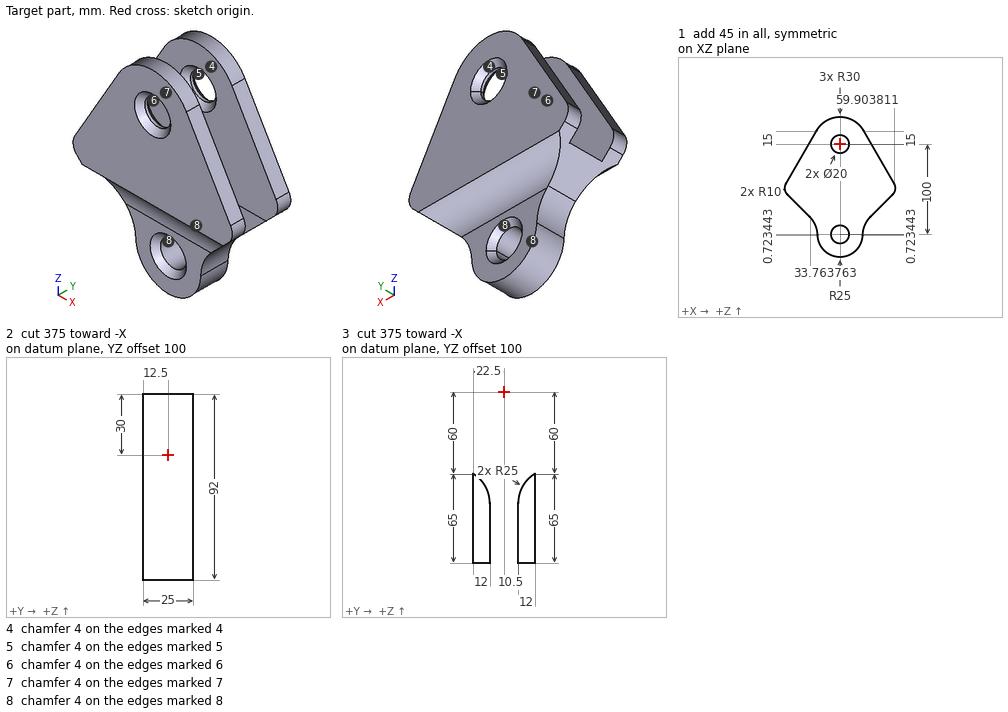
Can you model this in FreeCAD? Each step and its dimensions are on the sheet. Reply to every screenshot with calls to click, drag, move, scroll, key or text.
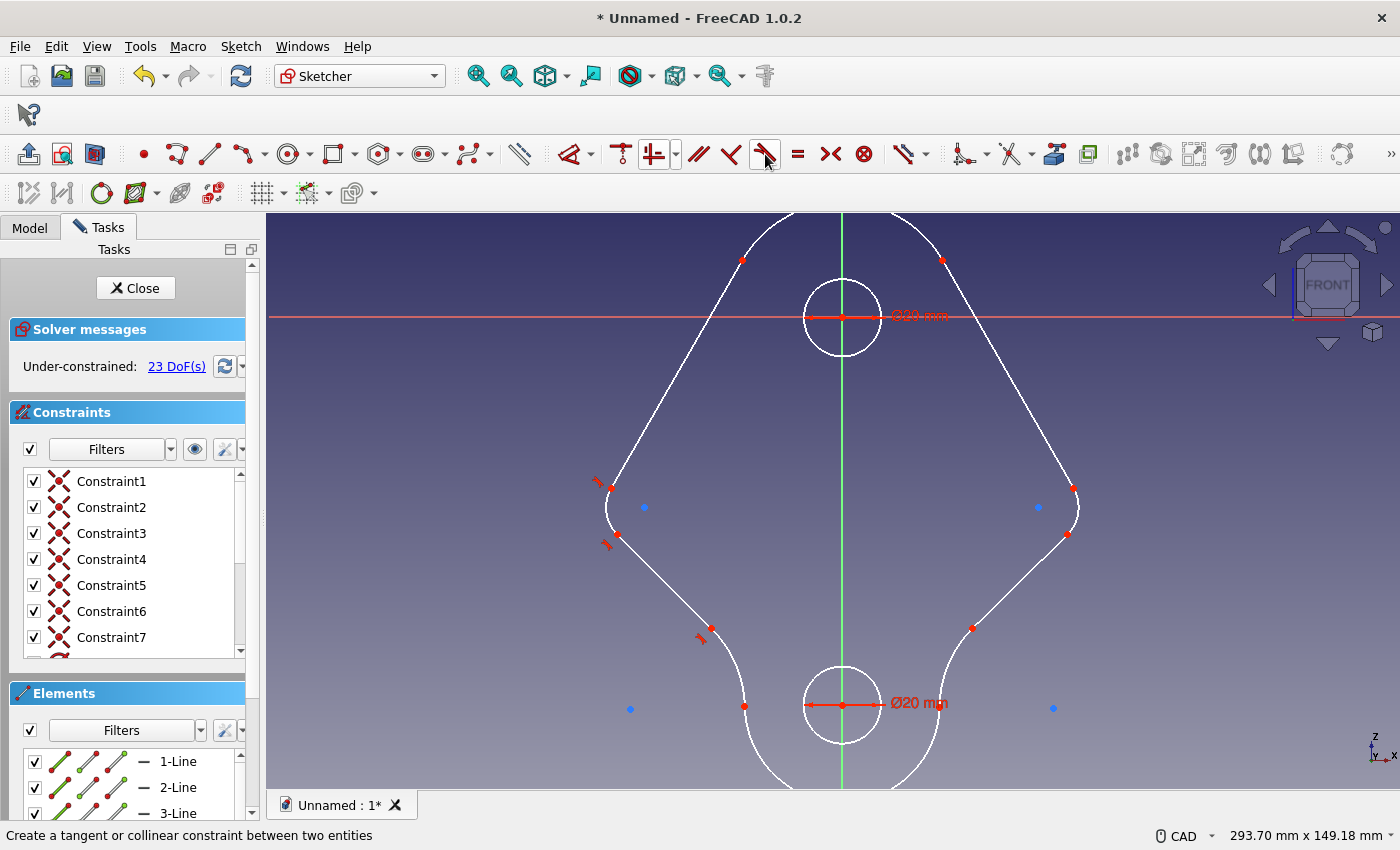
click(651, 420)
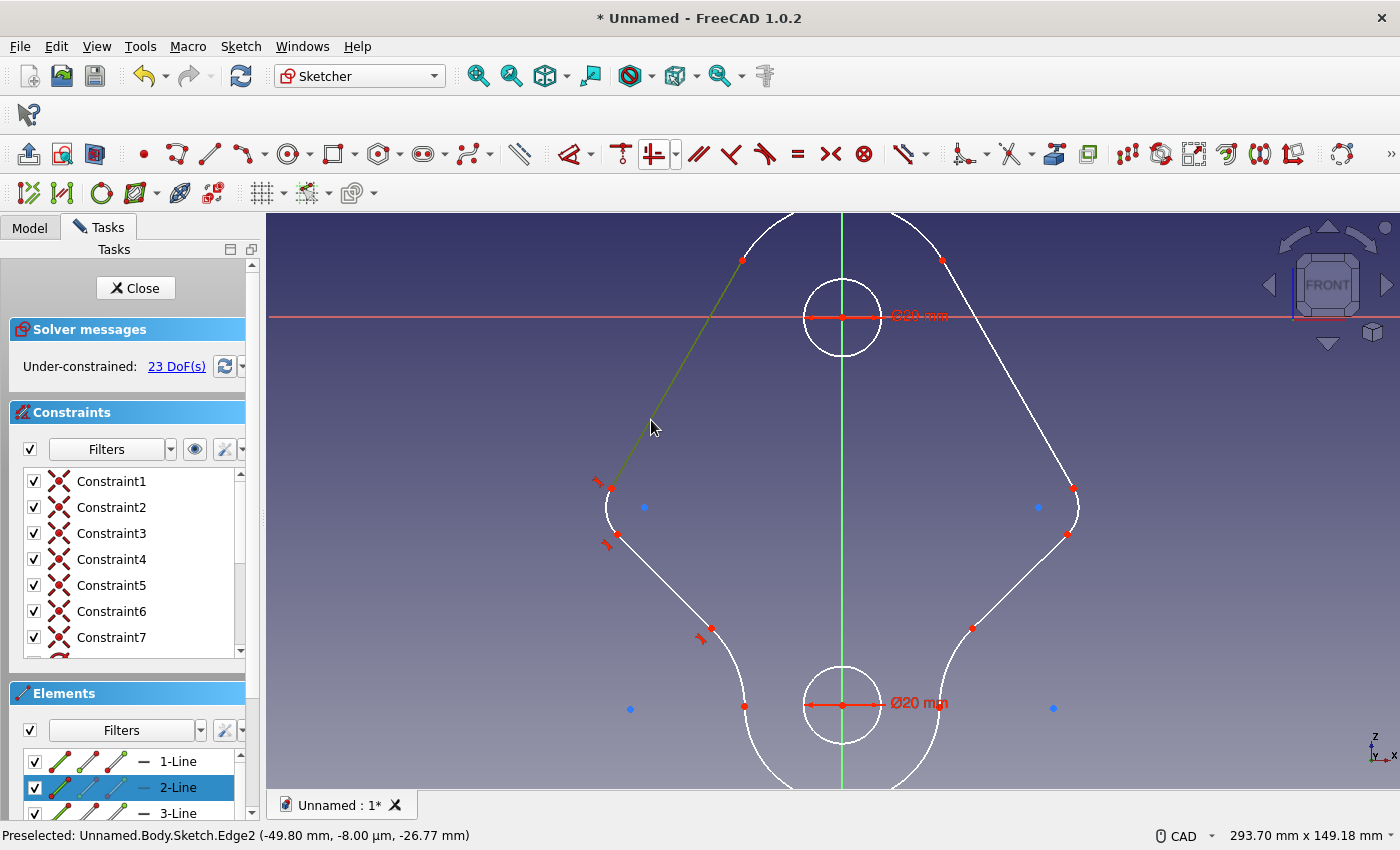
scroll(606, 502, down, 2)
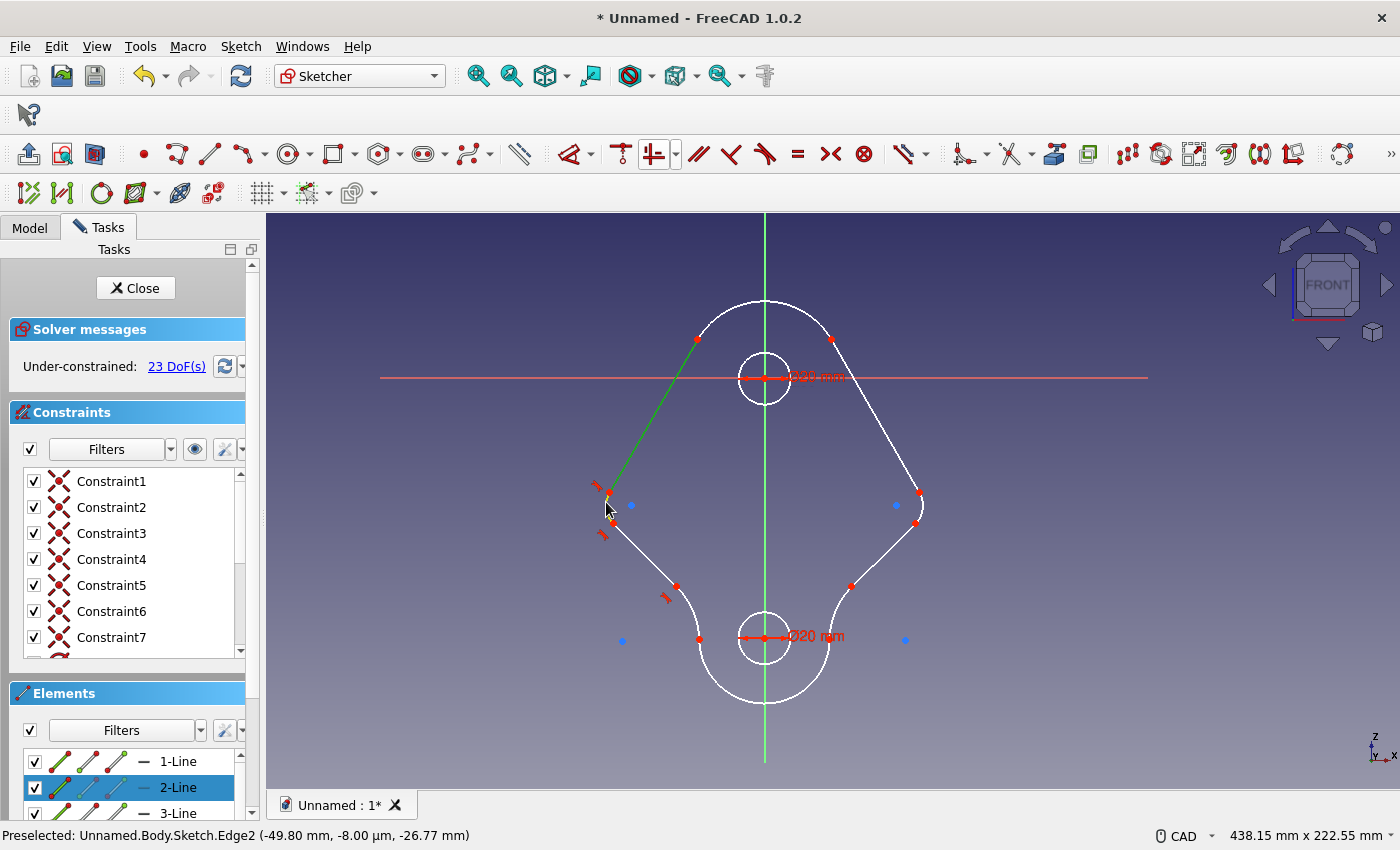
click(796, 308)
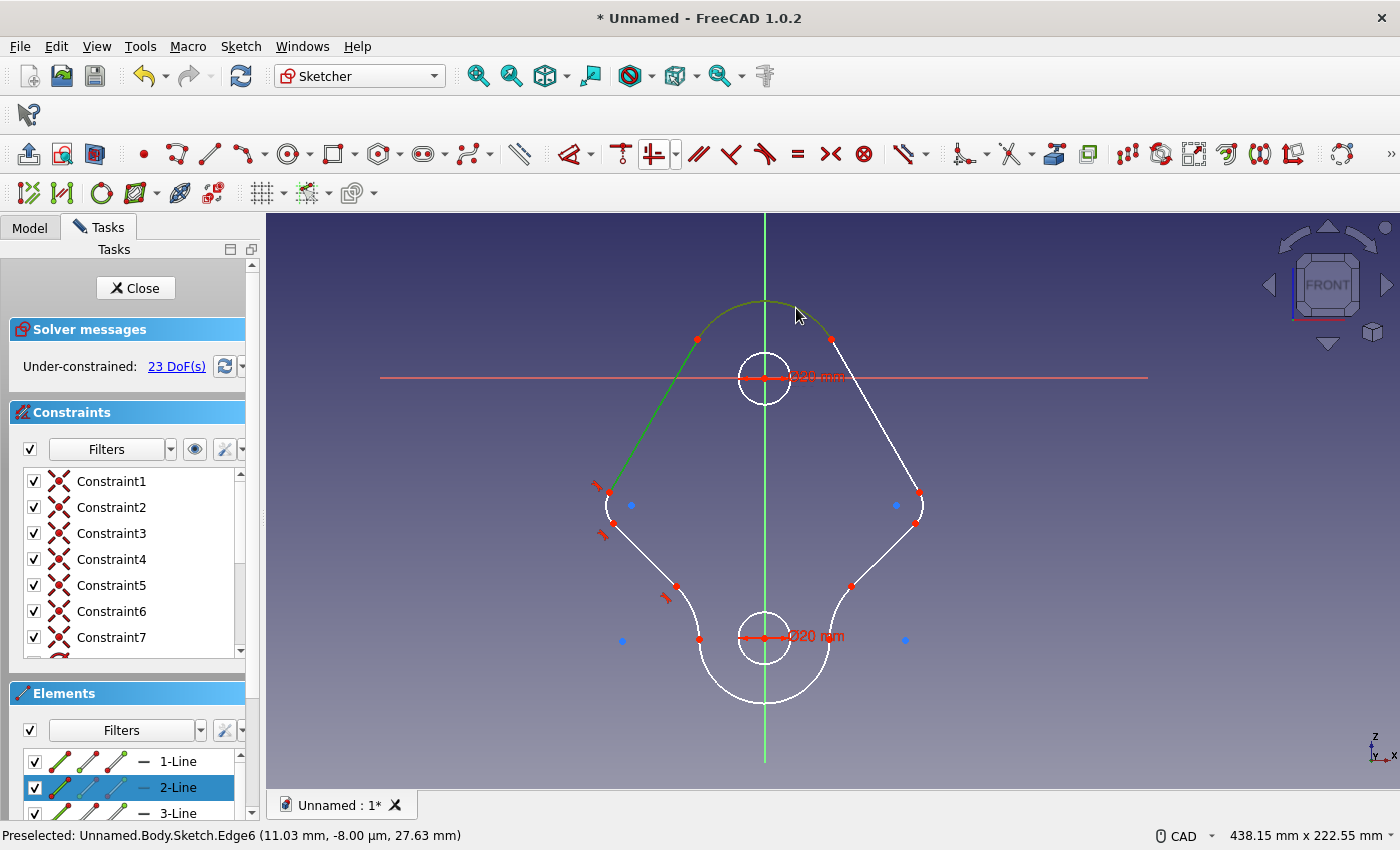
click(765, 154)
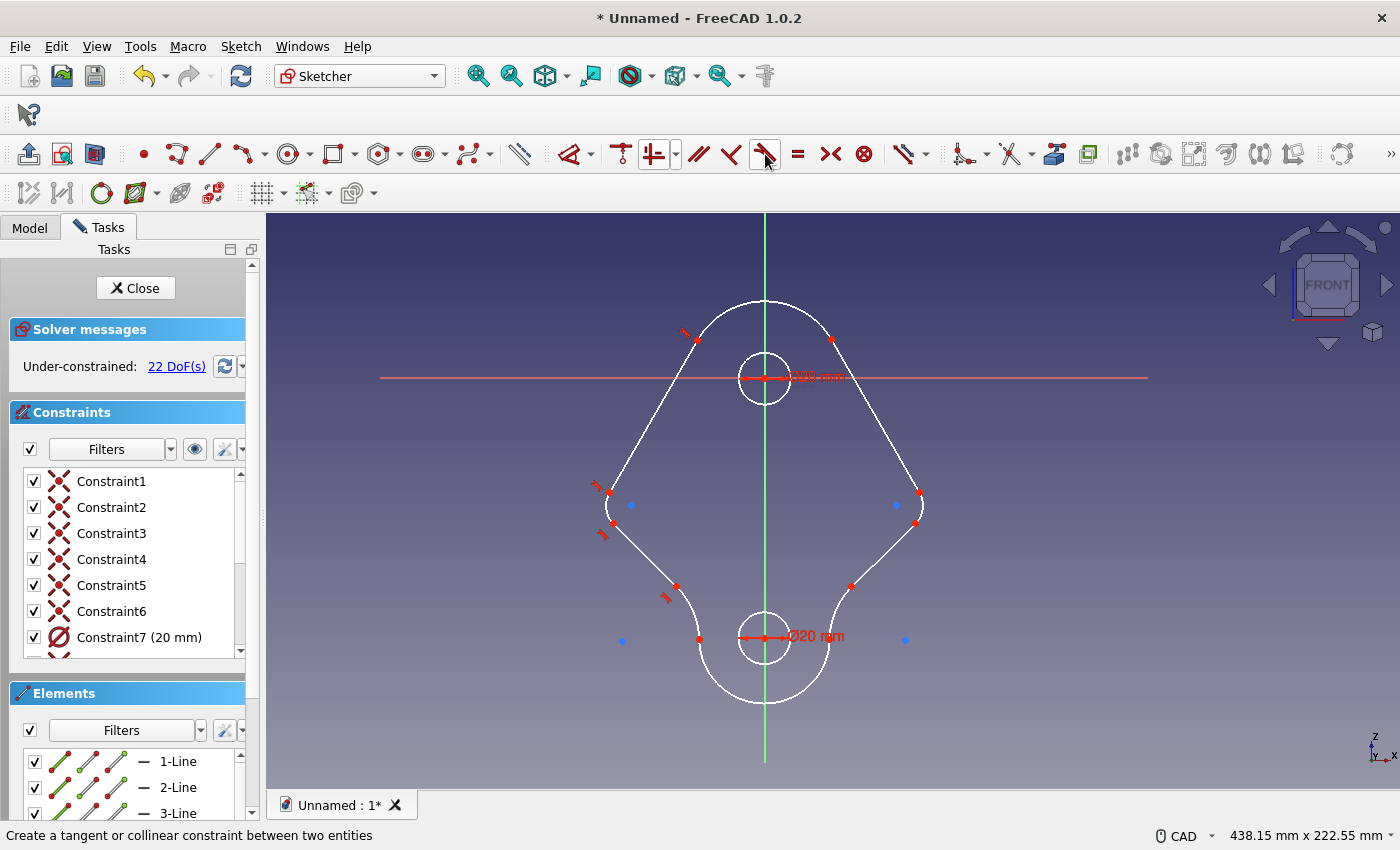
click(893, 447)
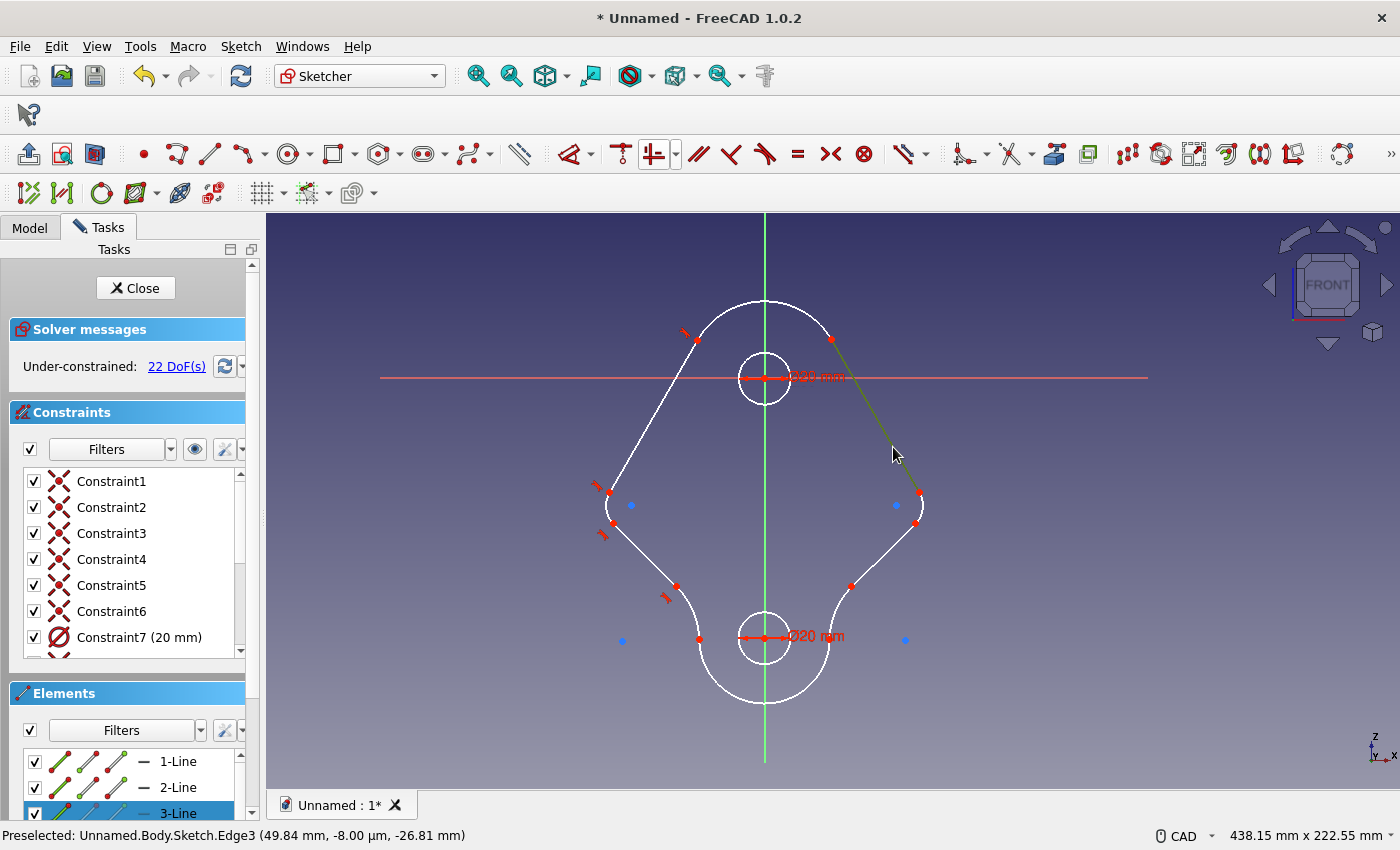
click(796, 308)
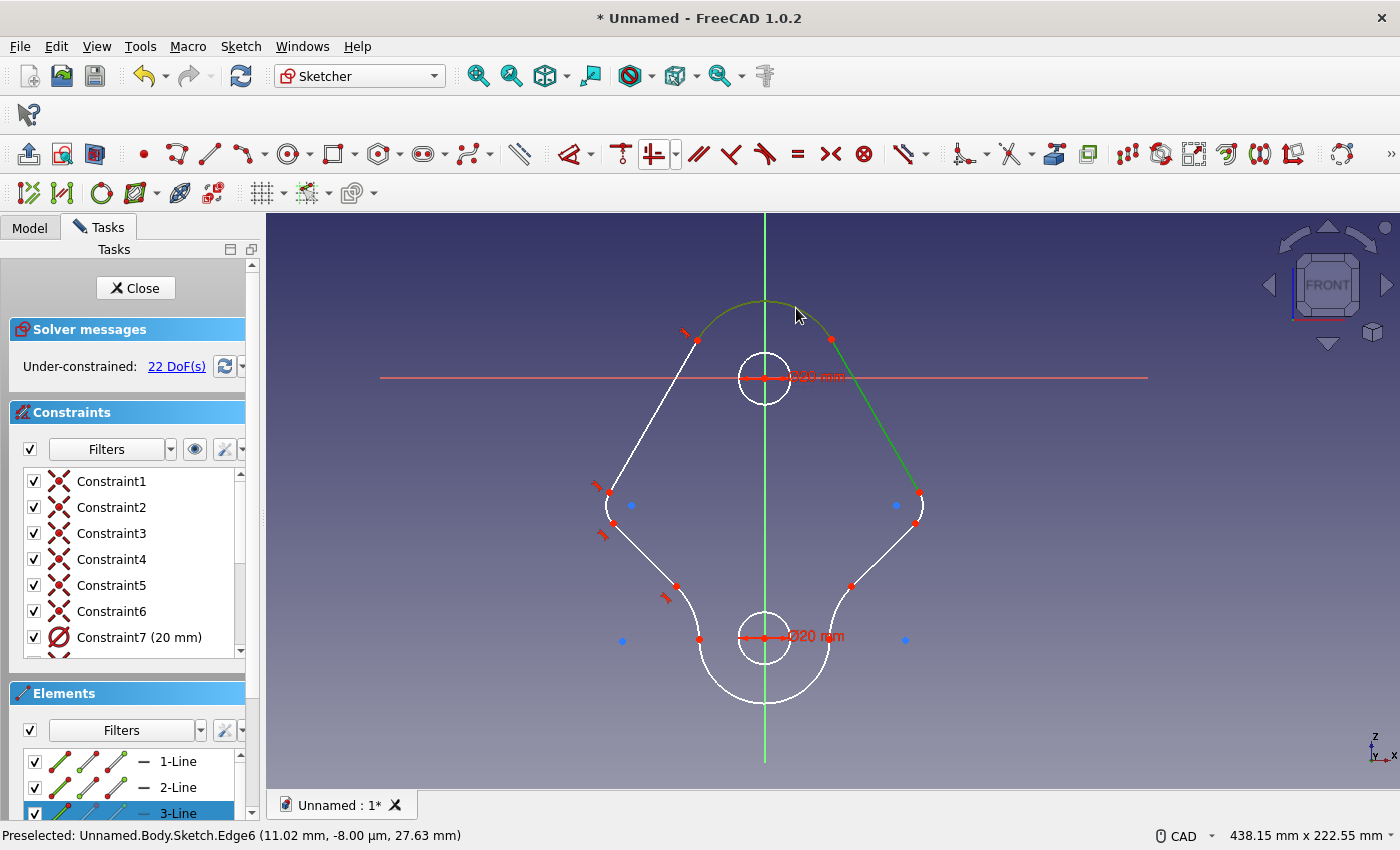
click(765, 154)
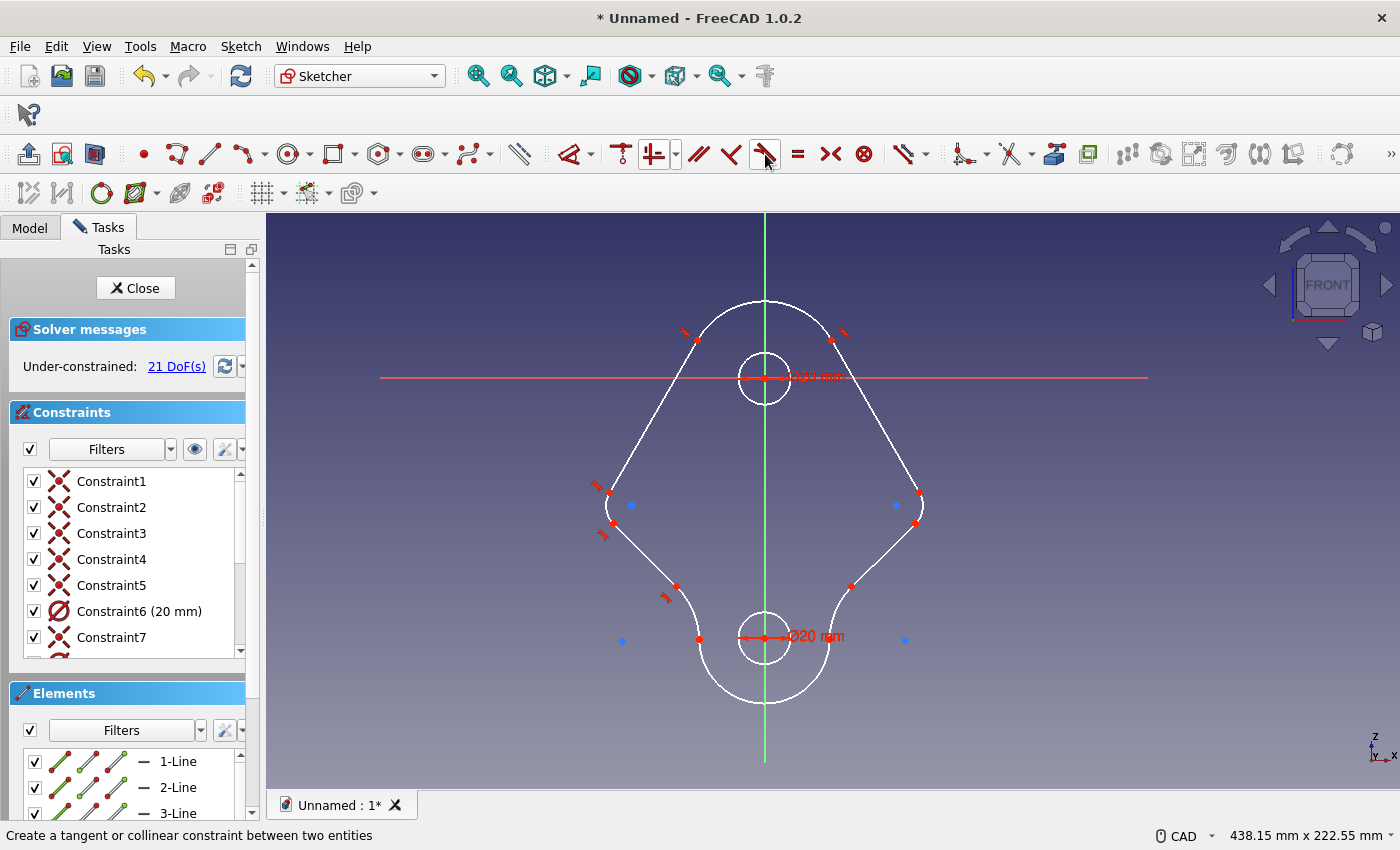
click(893, 447)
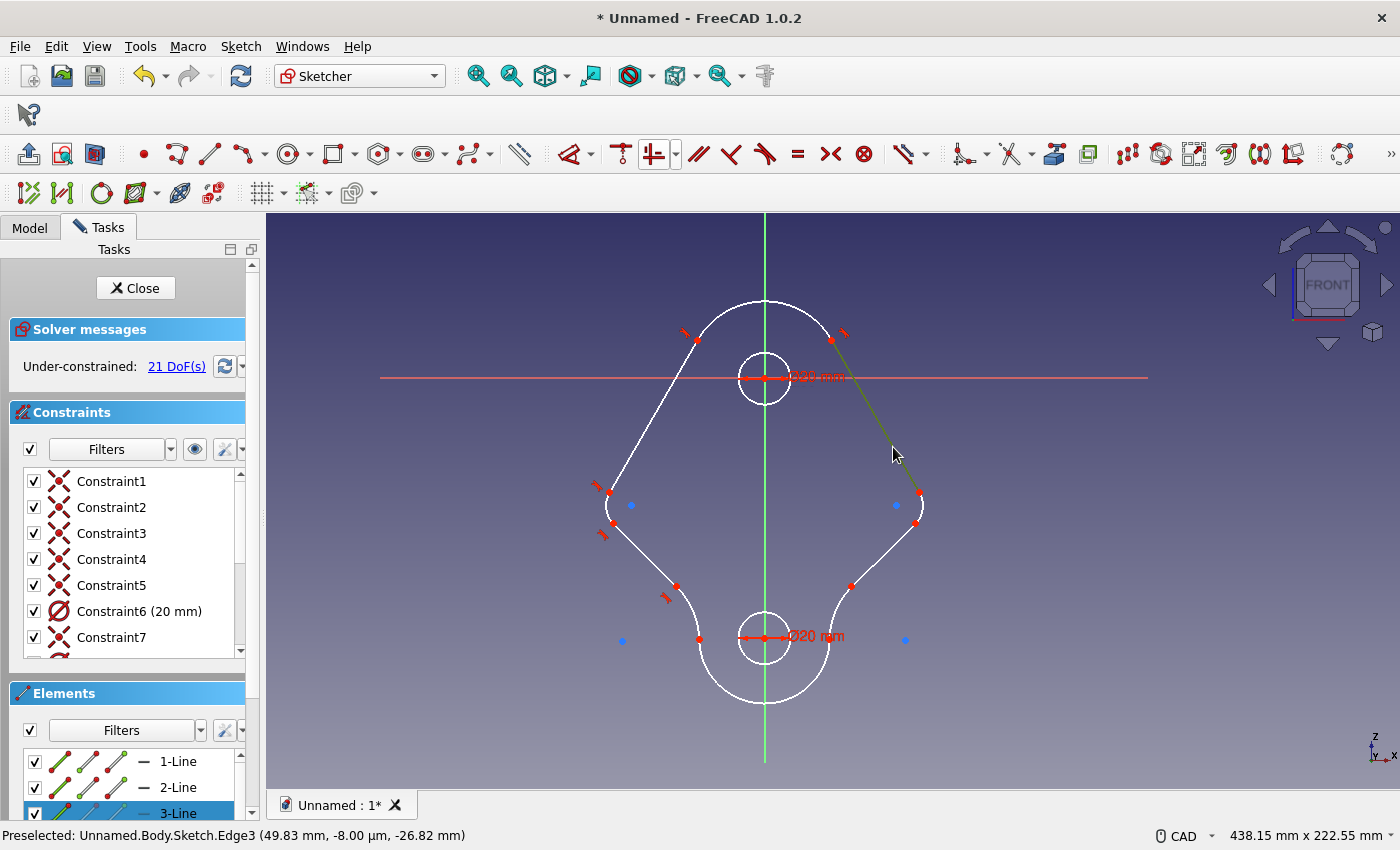
scroll(921, 516, up, 2)